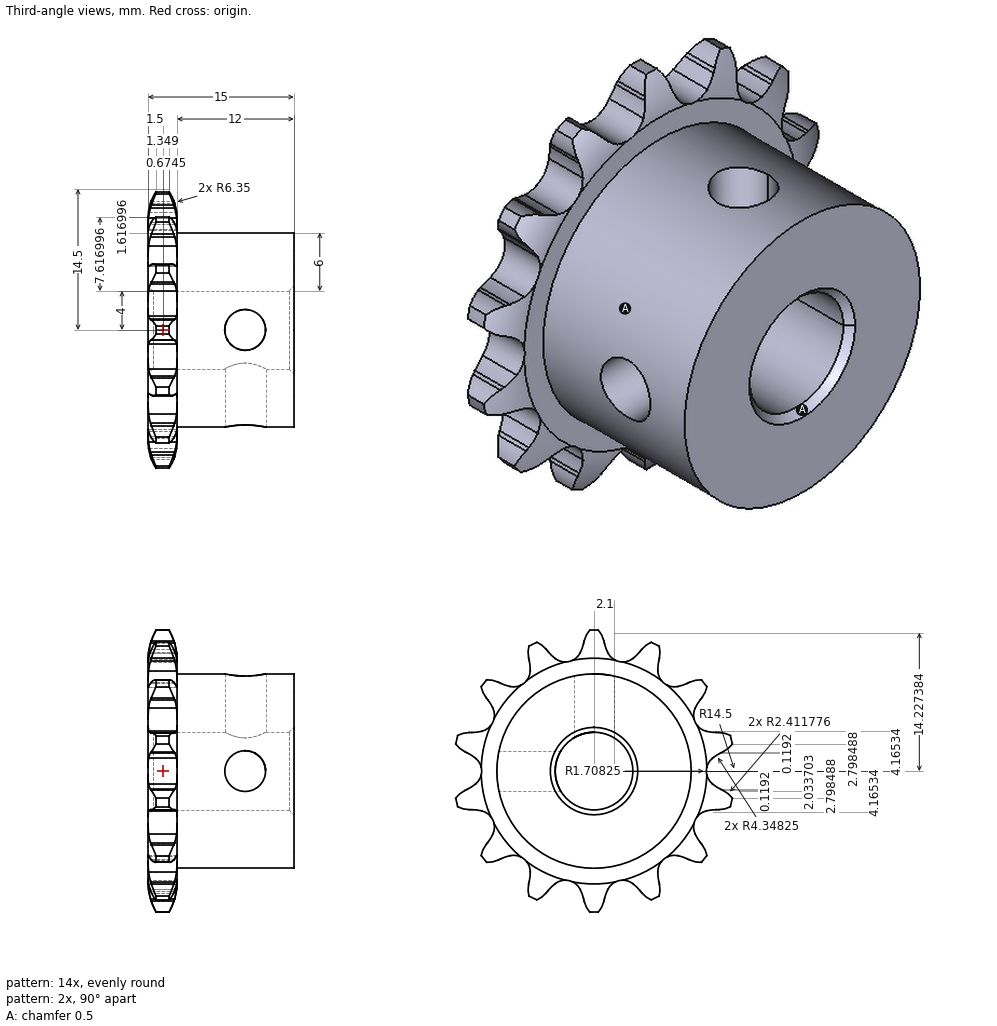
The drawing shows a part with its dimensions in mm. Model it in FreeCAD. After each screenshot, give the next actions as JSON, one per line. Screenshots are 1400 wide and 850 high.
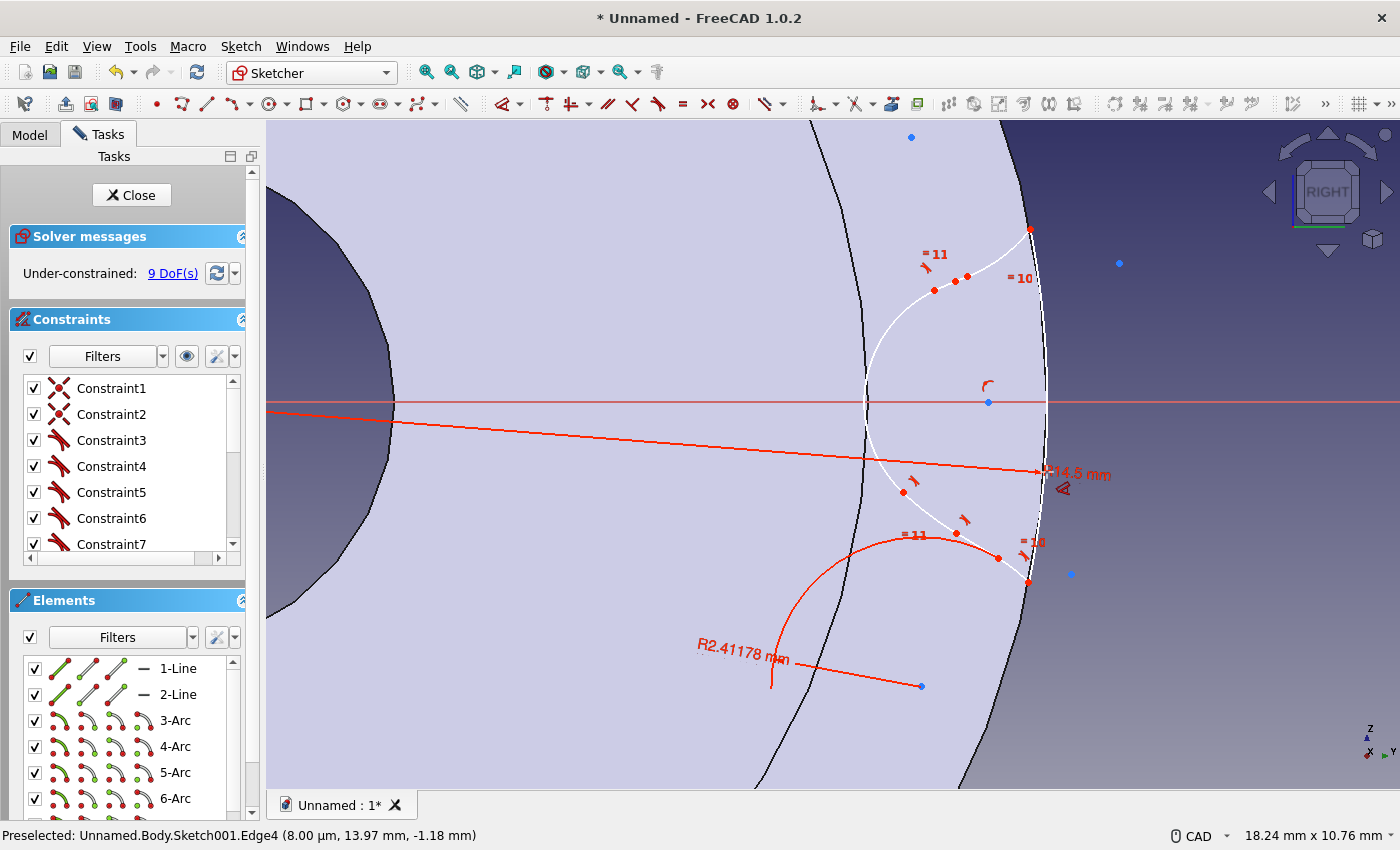
{"action": "left_click", "coordinate": [944, 286]}
{"action": "left_click", "coordinate": [931, 257]}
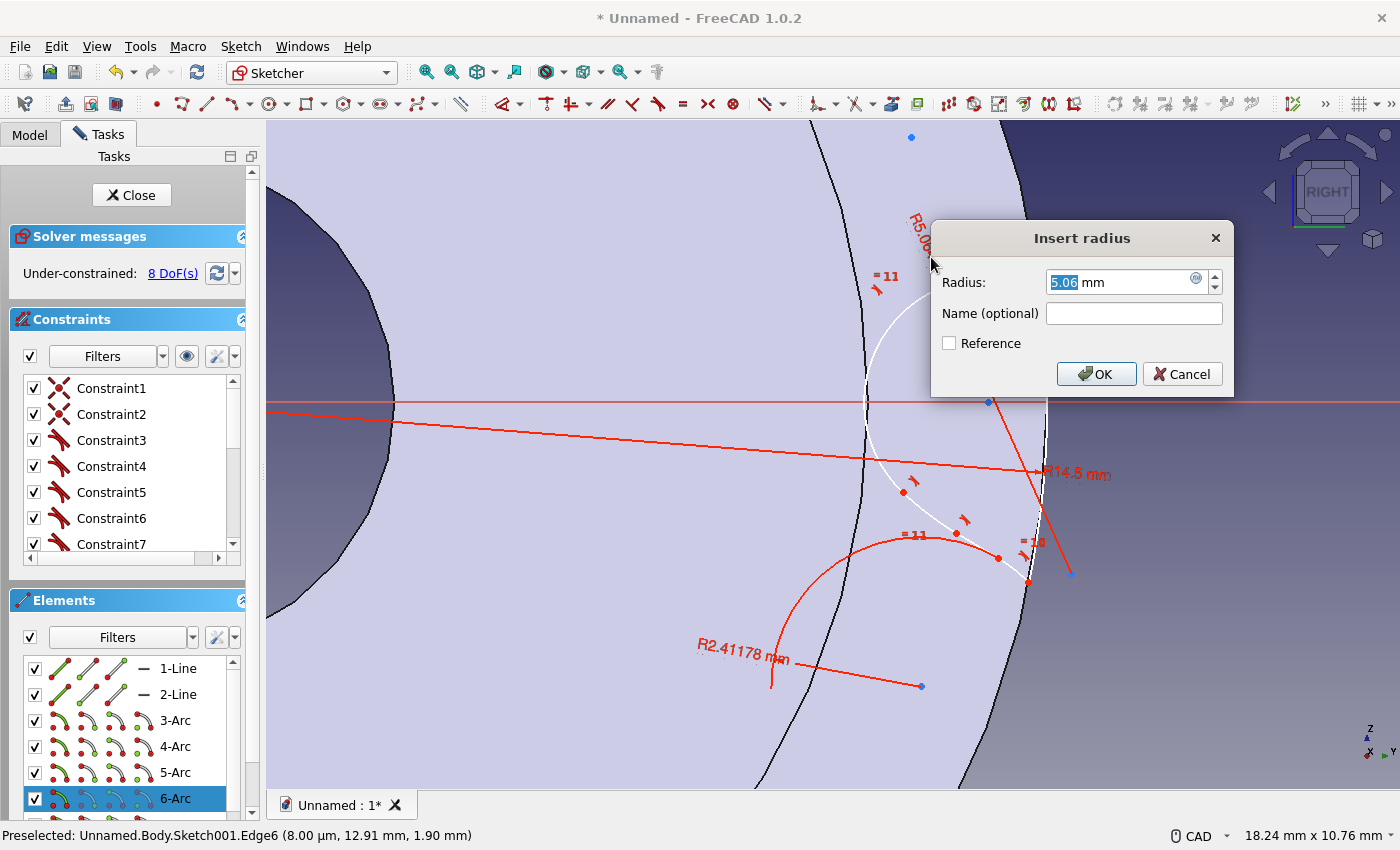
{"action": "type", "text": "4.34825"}
{"action": "key", "text": "Return"}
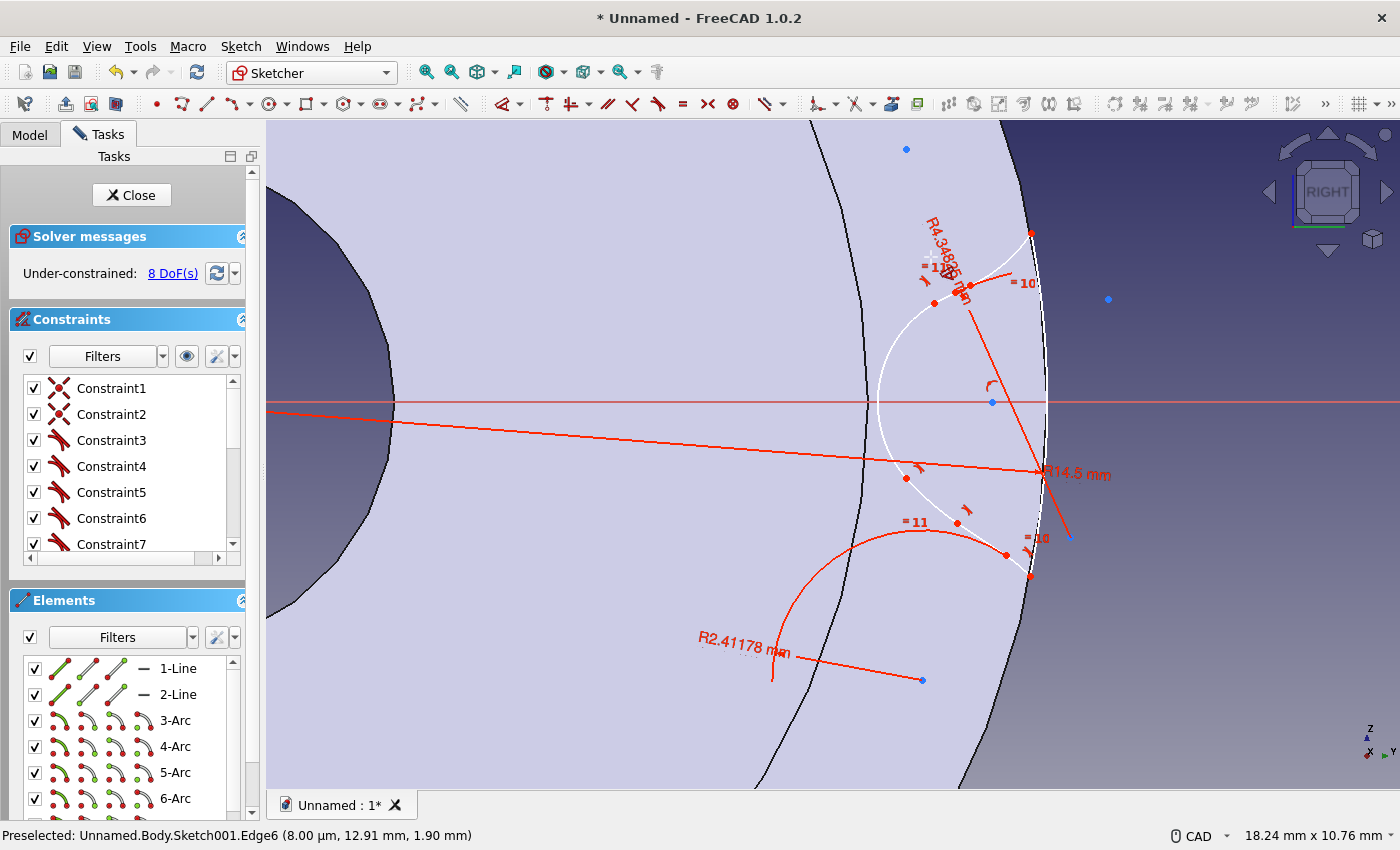
{"action": "left_click", "coordinate": [893, 346]}
{"action": "left_click", "coordinate": [865, 330]}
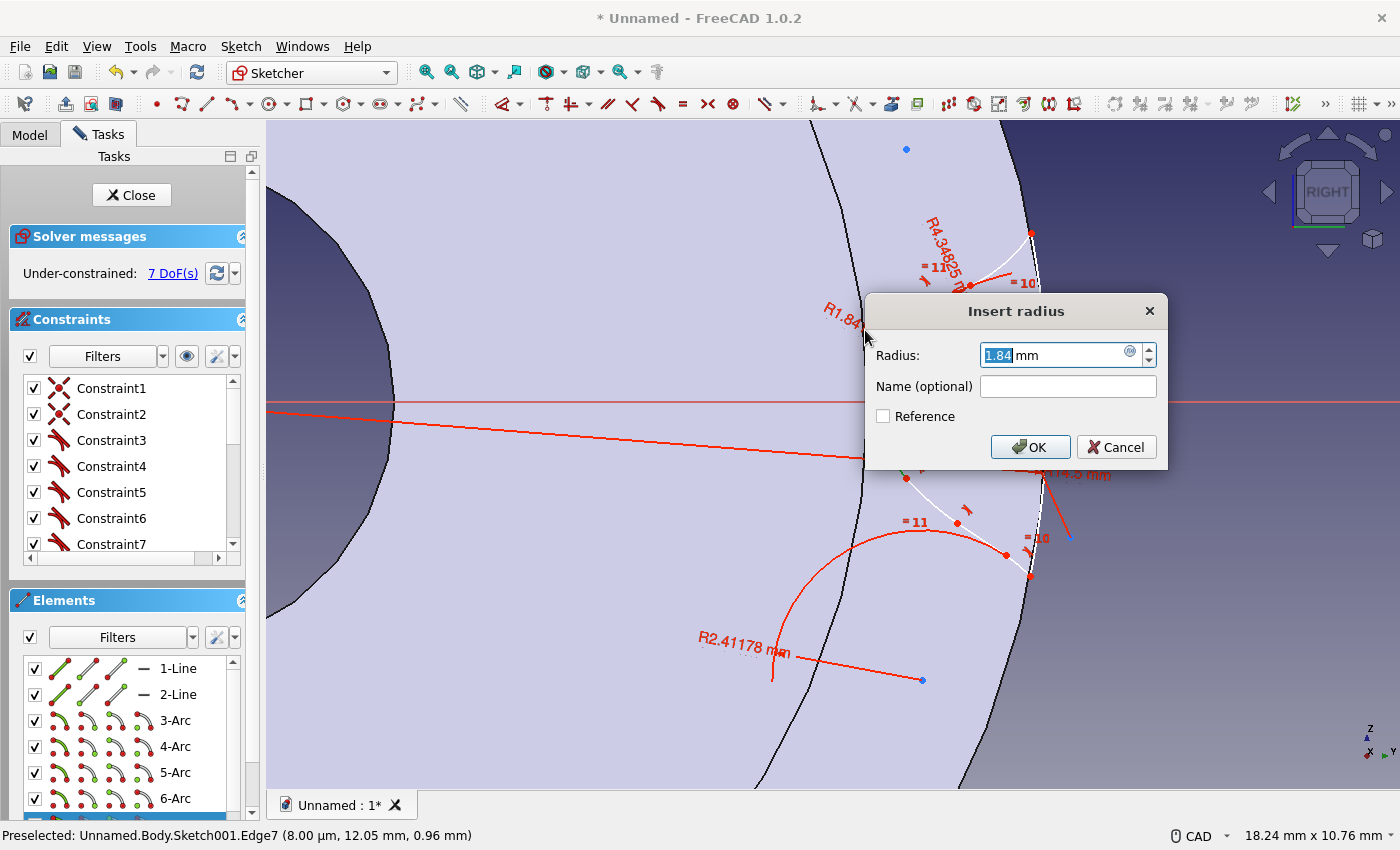
{"action": "type", "text": "1.70825"}
{"action": "key", "text": "Return"}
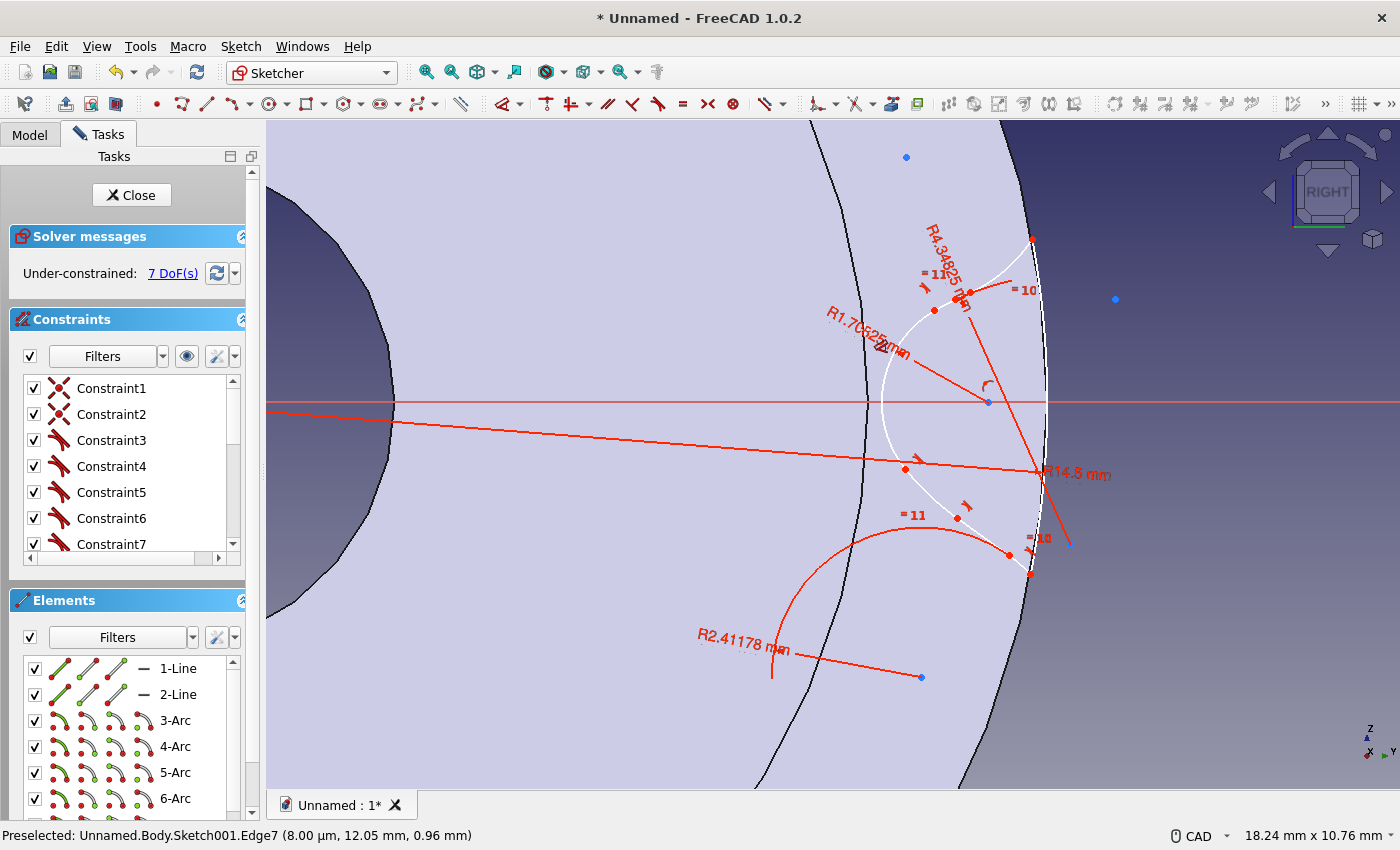
{"action": "scroll", "coordinate": [973, 530], "scroll_direction": "up", "scroll_amount": 9}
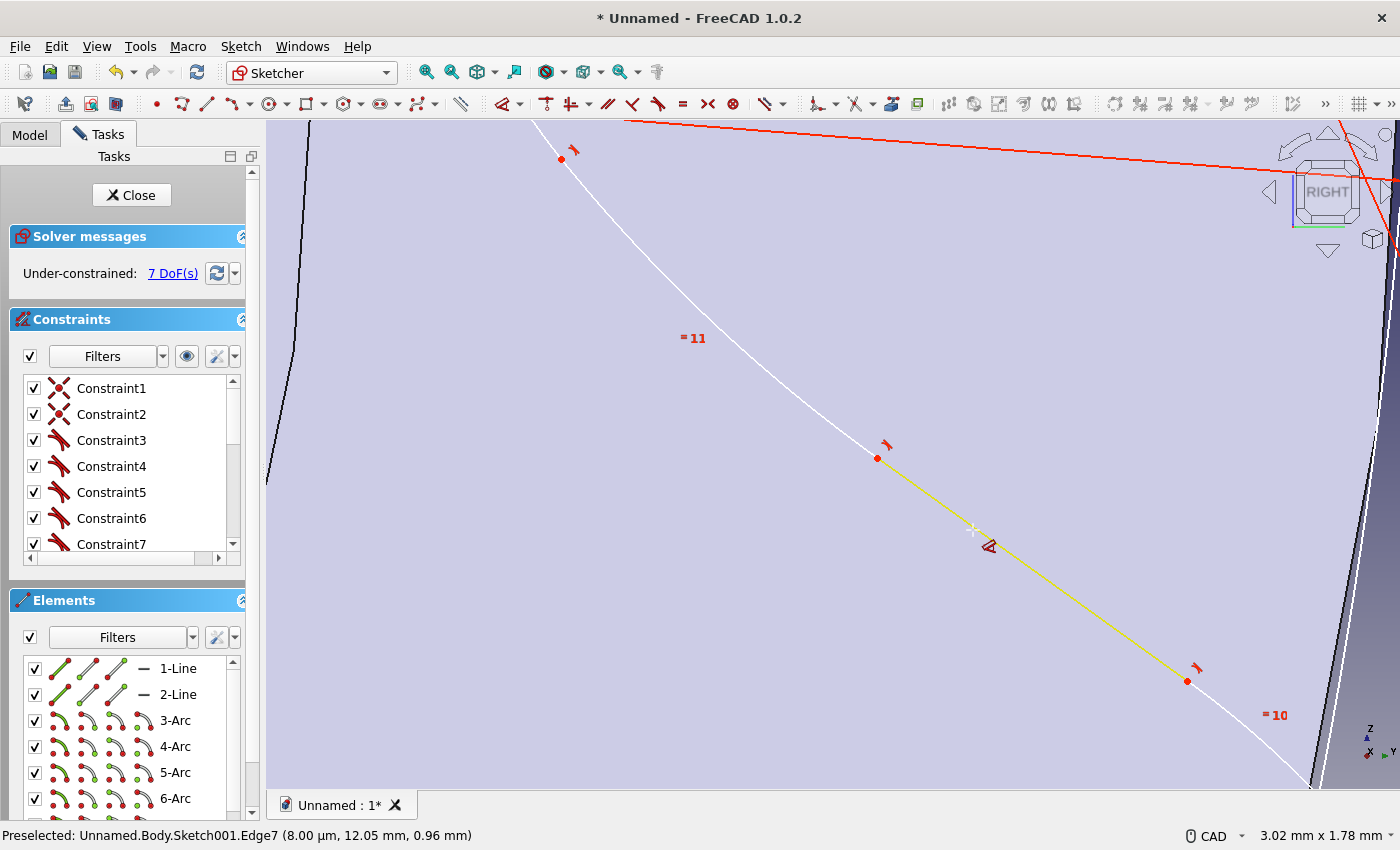
{"action": "left_click", "coordinate": [971, 525]}
{"action": "left_click", "coordinate": [1222, 570]}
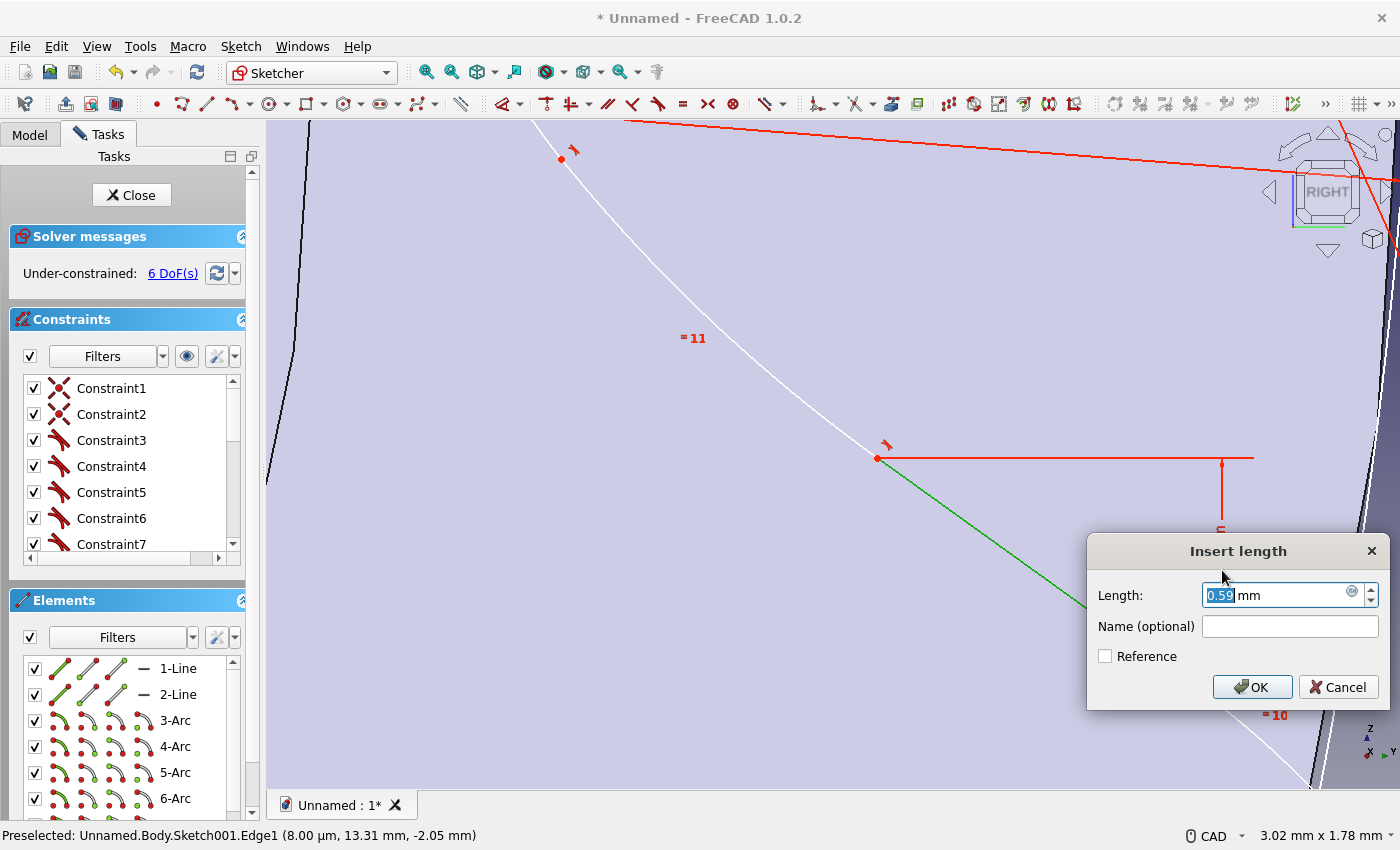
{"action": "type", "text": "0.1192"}
{"action": "key", "text": "Return"}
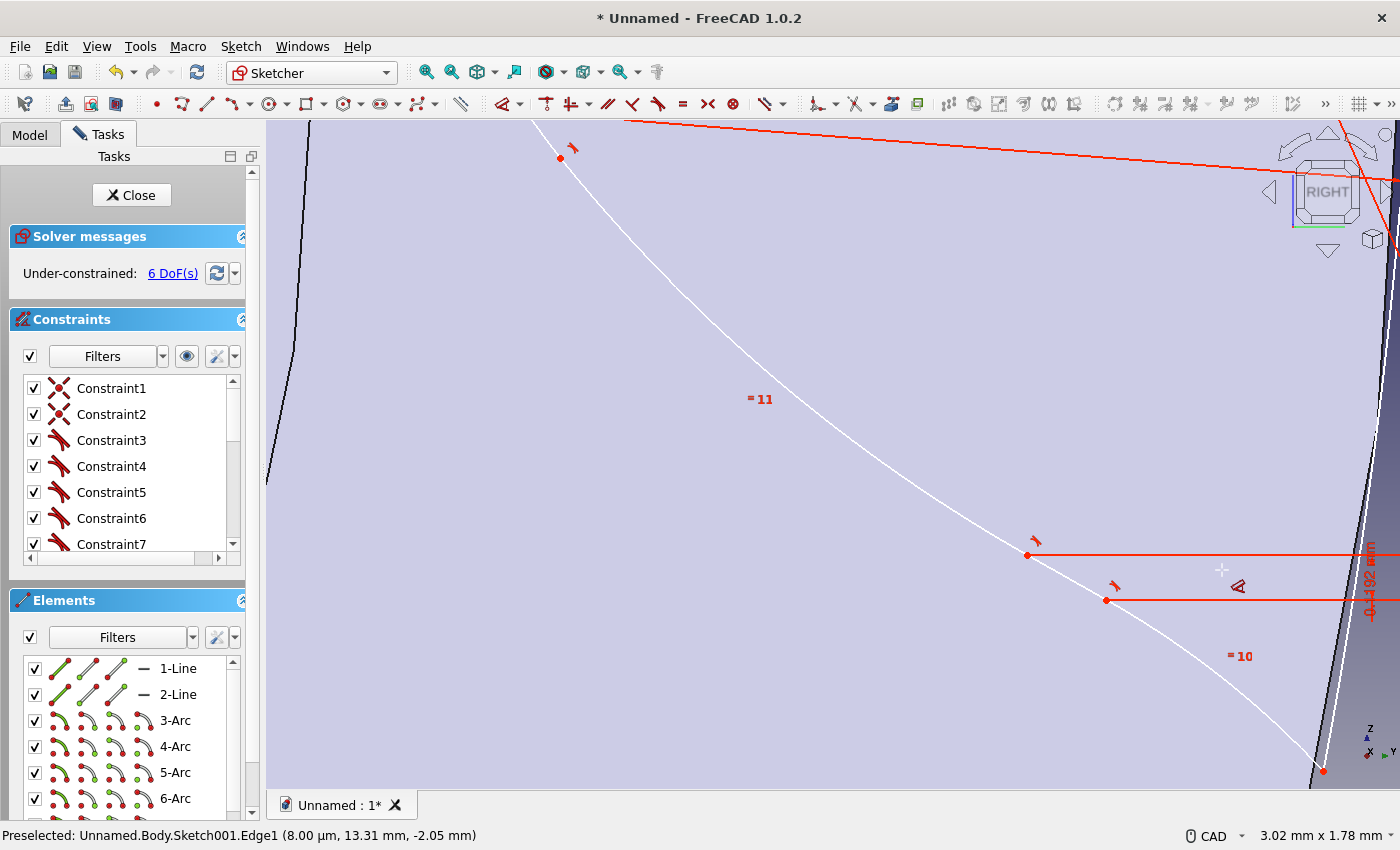
{"action": "scroll", "coordinate": [739, 631], "scroll_direction": "down", "scroll_amount": 8}